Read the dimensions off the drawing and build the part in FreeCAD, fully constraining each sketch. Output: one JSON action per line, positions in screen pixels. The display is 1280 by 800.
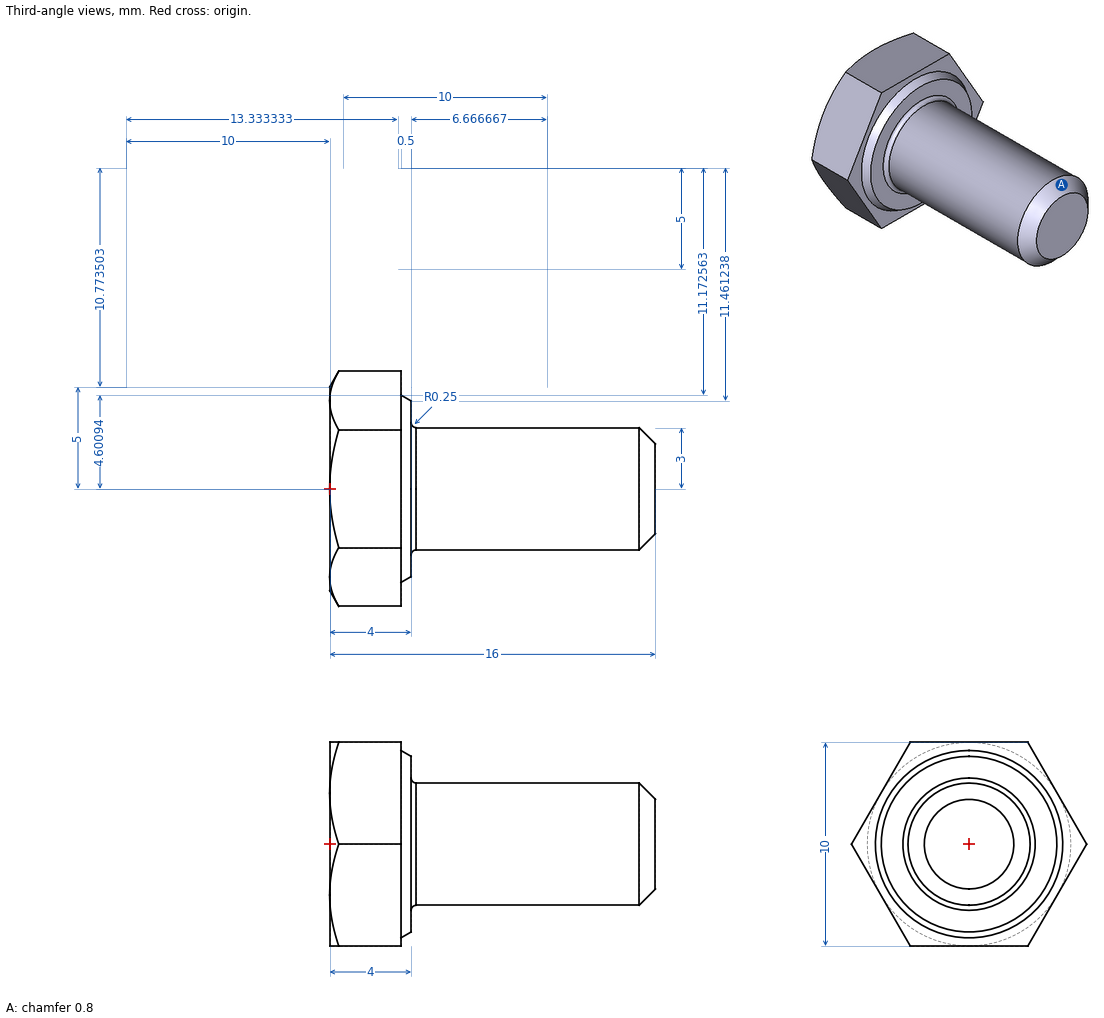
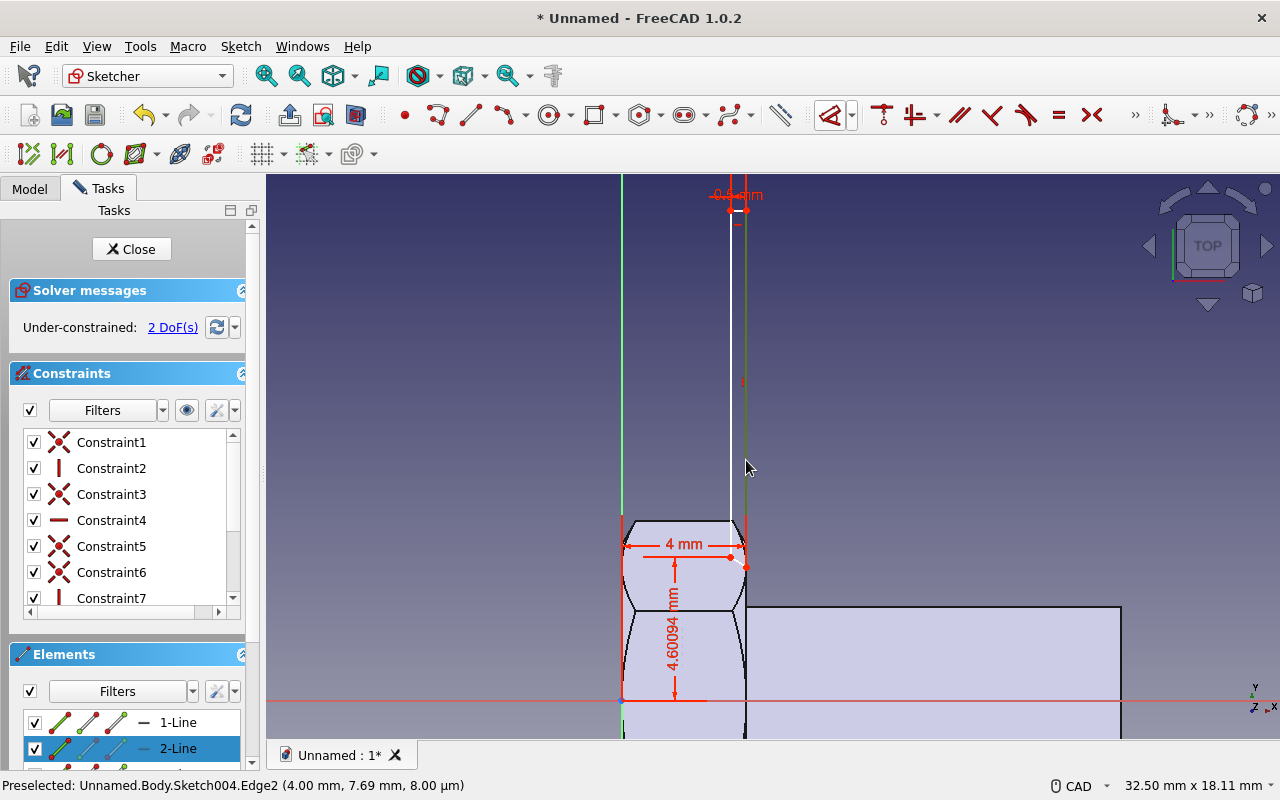
{"action": "key", "text": "i"}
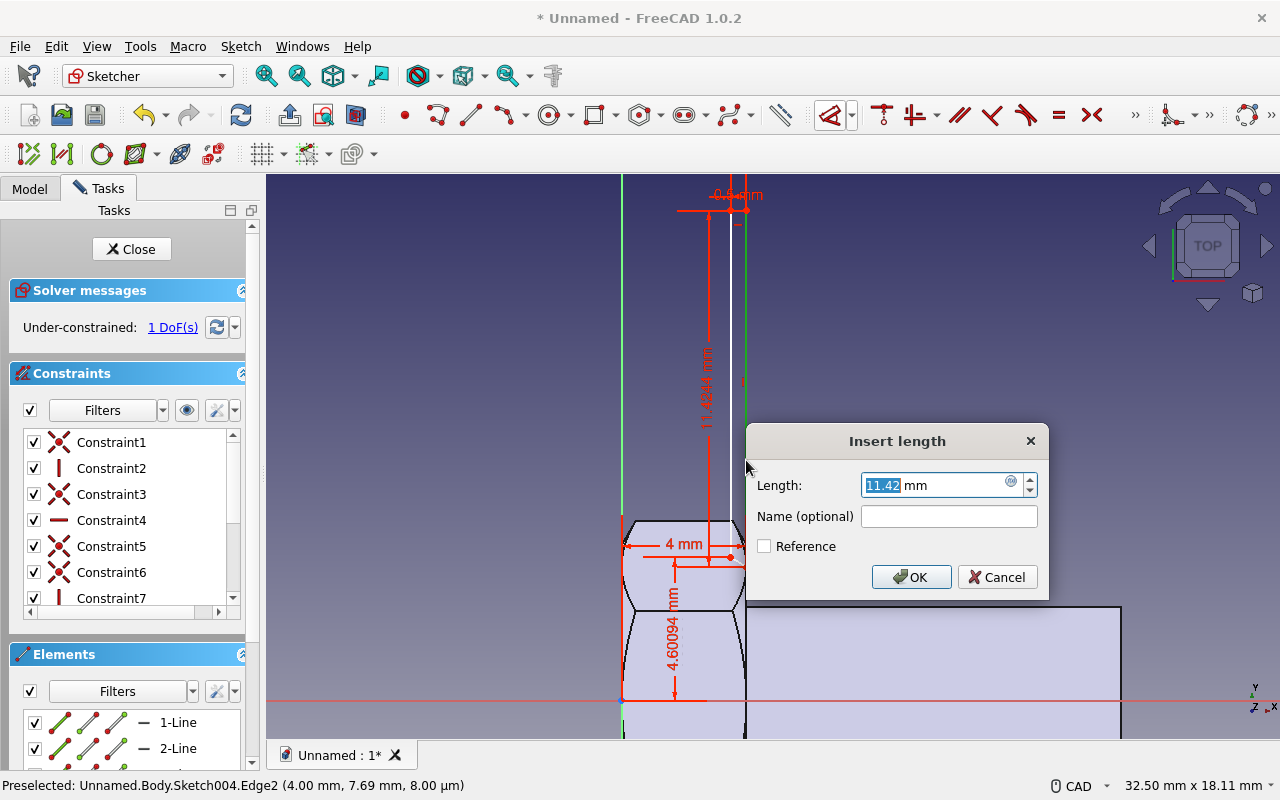
{"action": "type", "text": "11.461238"}
{"action": "key", "text": "Return"}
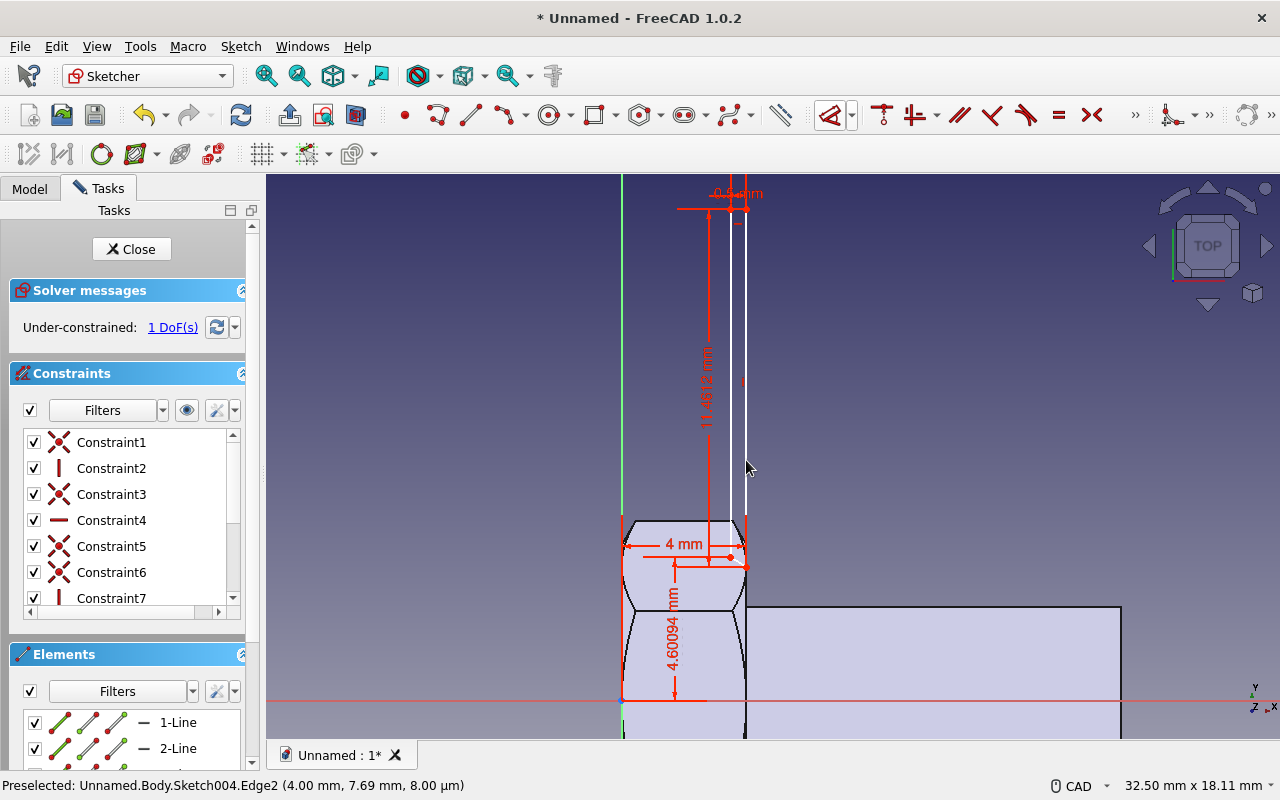
{"action": "left_click", "coordinate": [731, 314]}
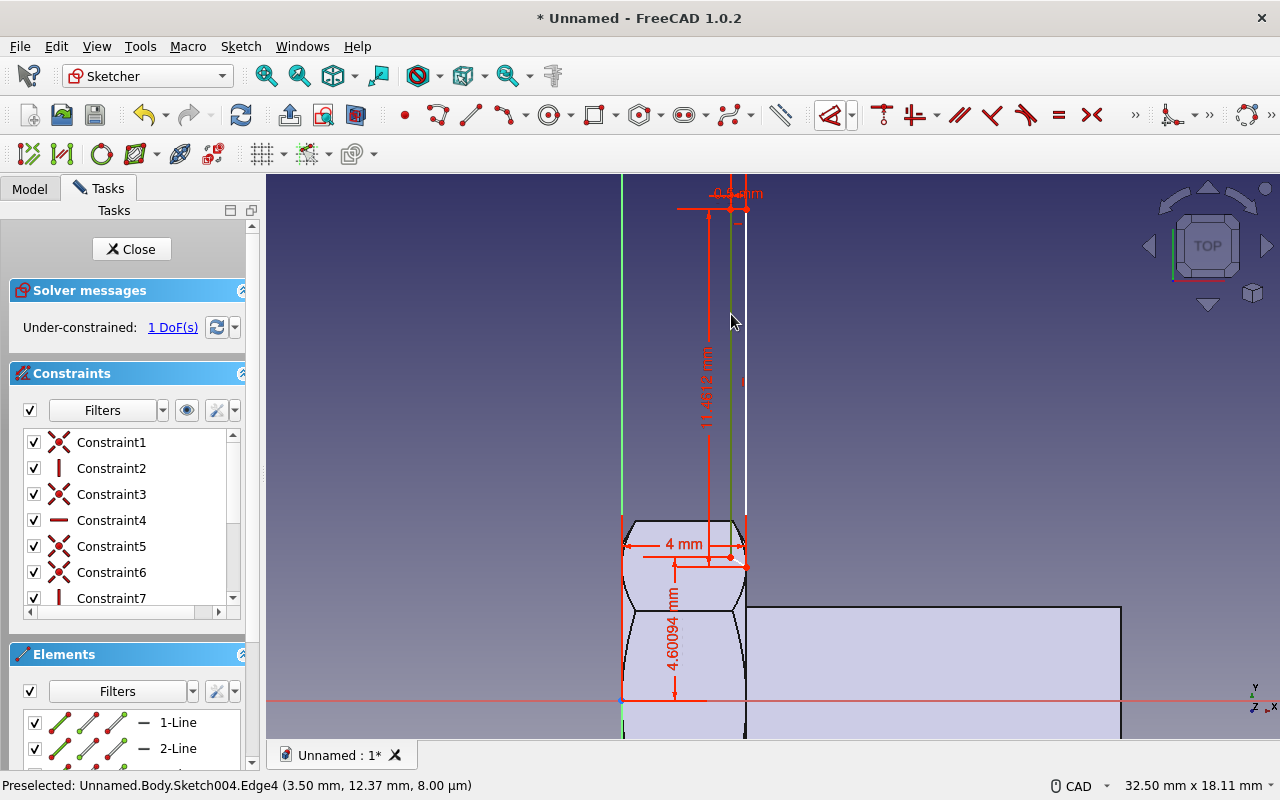
{"action": "left_click", "coordinate": [852, 116]}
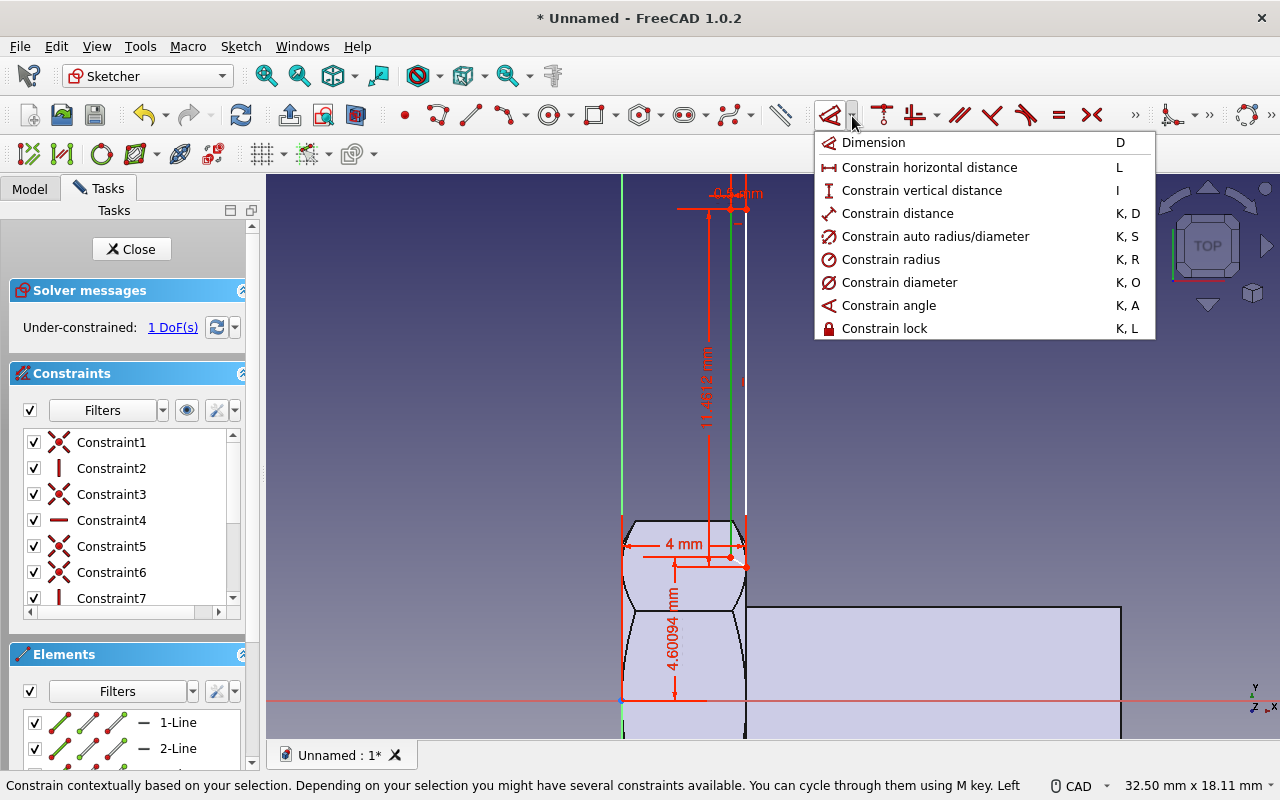
{"action": "left_click", "coordinate": [985, 190]}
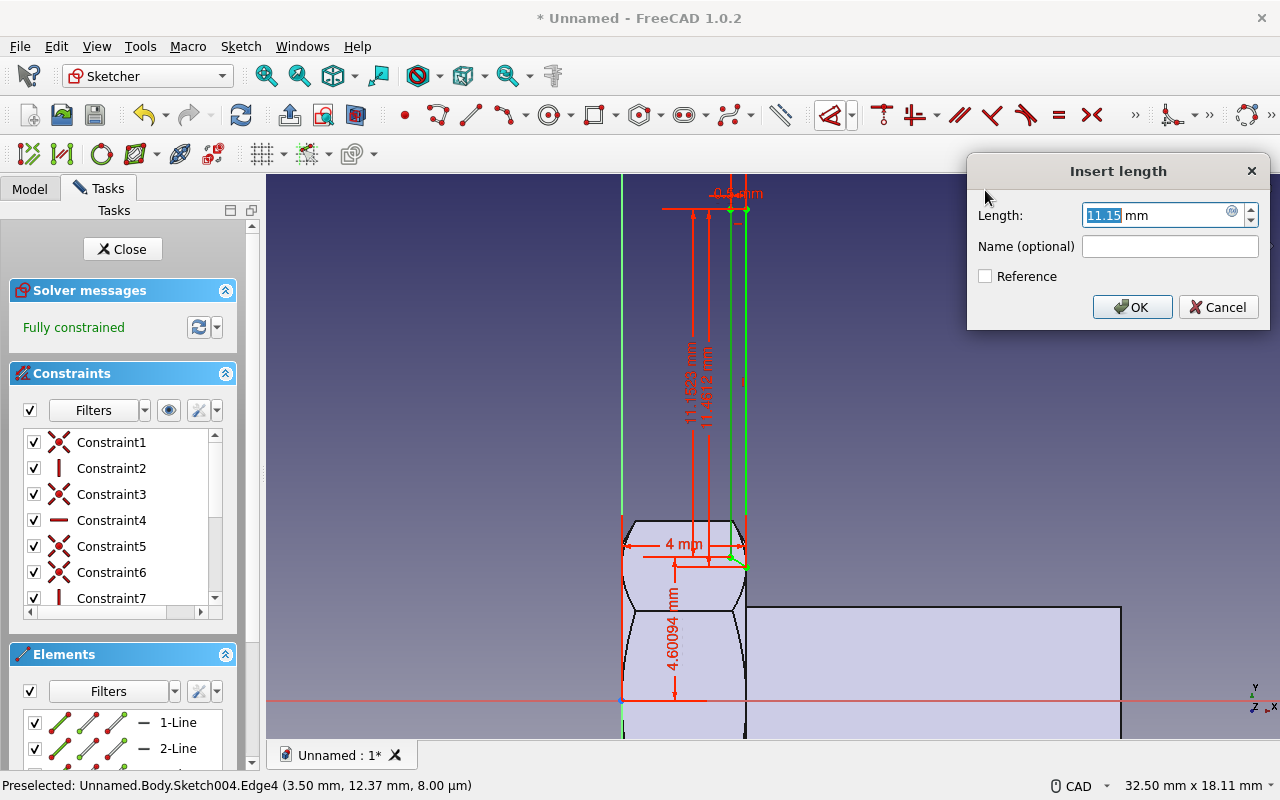
{"action": "type", "text": "11.172563"}
{"action": "key", "text": "Return"}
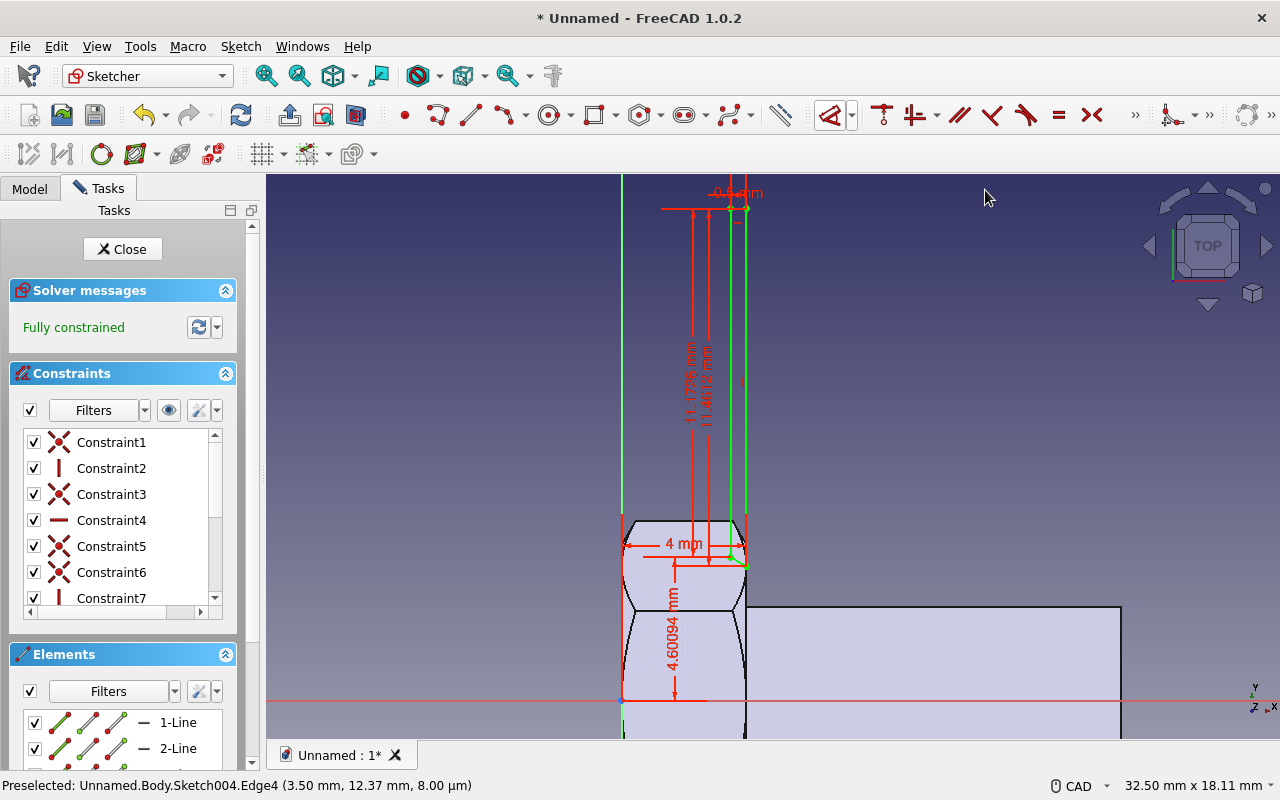
{"action": "left_click", "coordinate": [123, 249]}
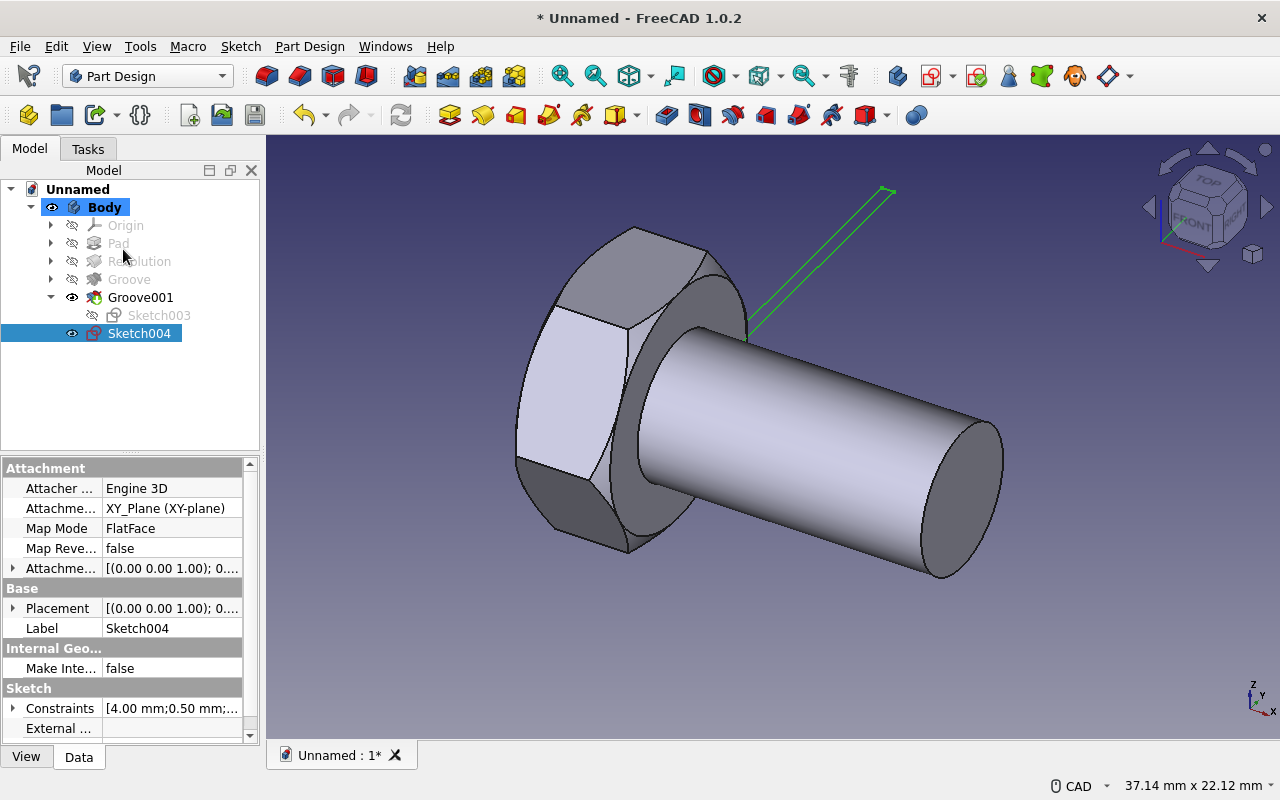
{"action": "left_click", "coordinate": [733, 116]}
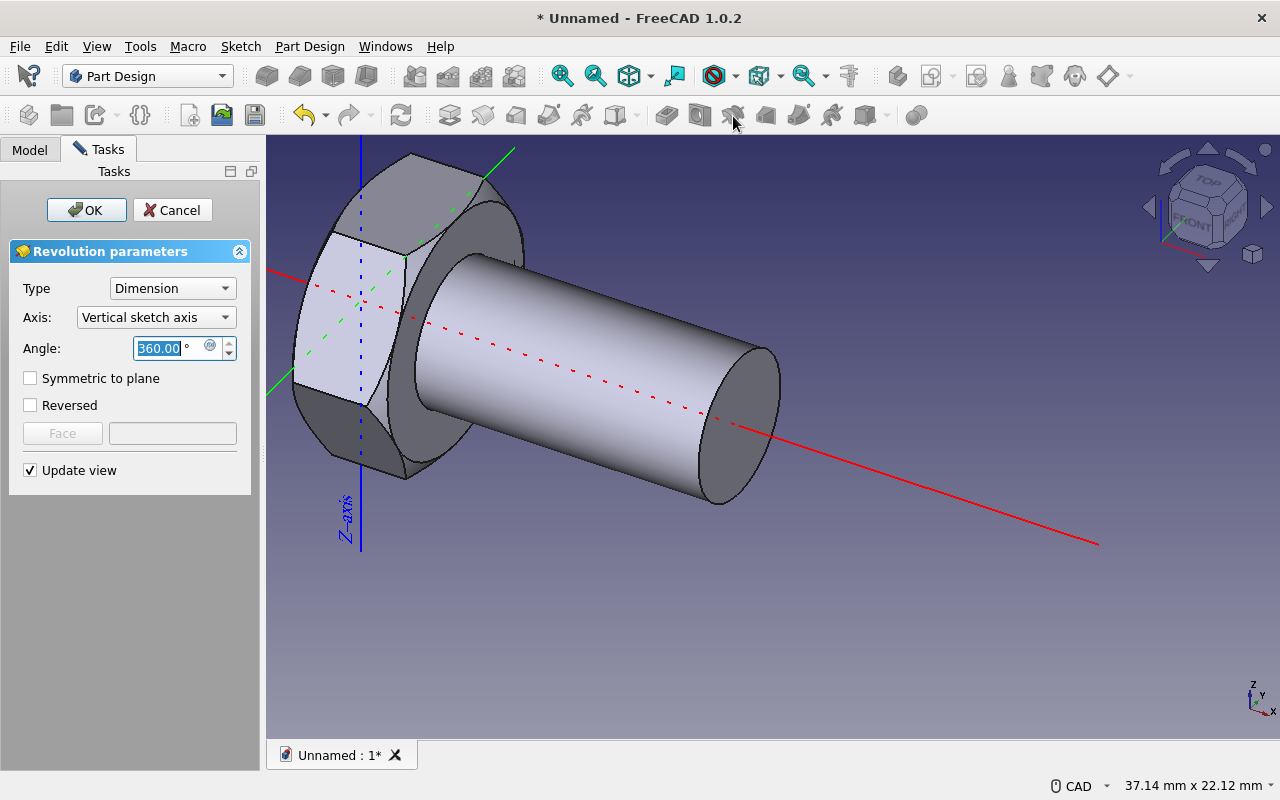
{"action": "left_click", "coordinate": [157, 318]}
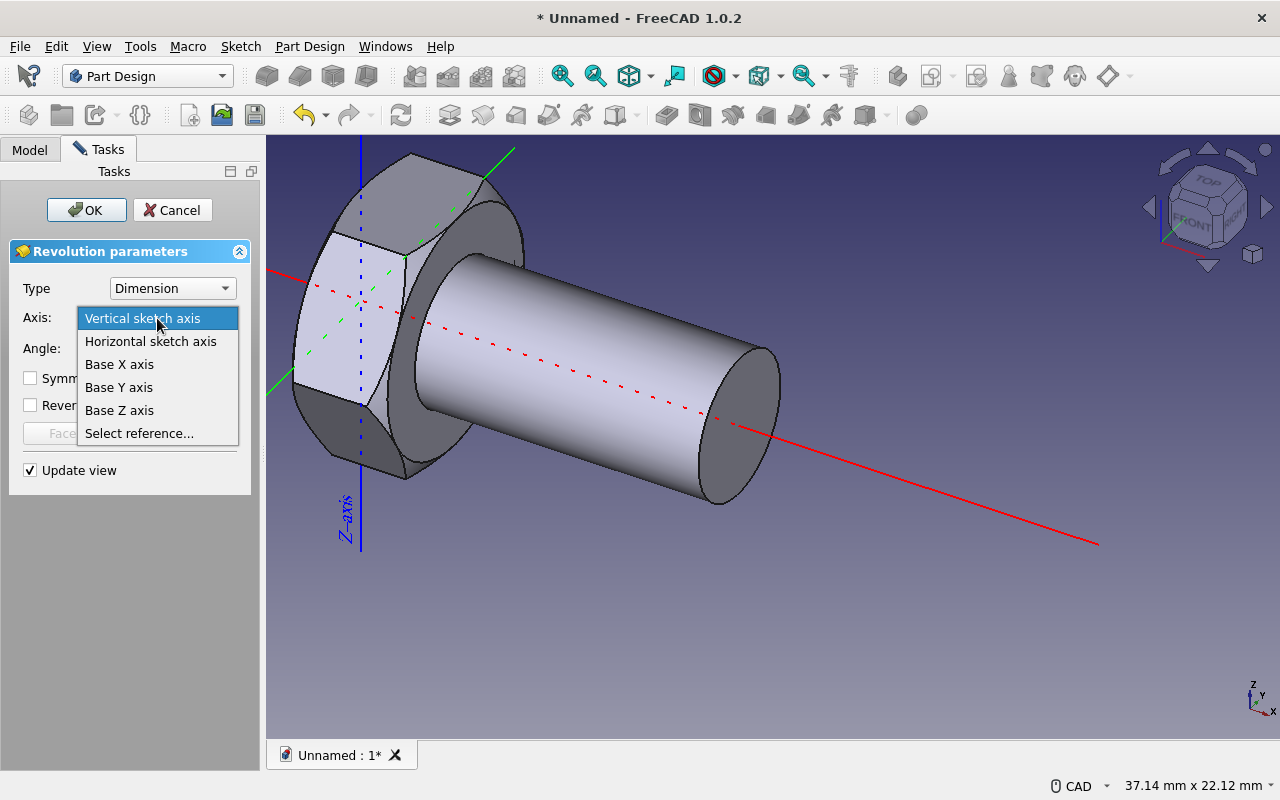
{"action": "left_click", "coordinate": [156, 342]}